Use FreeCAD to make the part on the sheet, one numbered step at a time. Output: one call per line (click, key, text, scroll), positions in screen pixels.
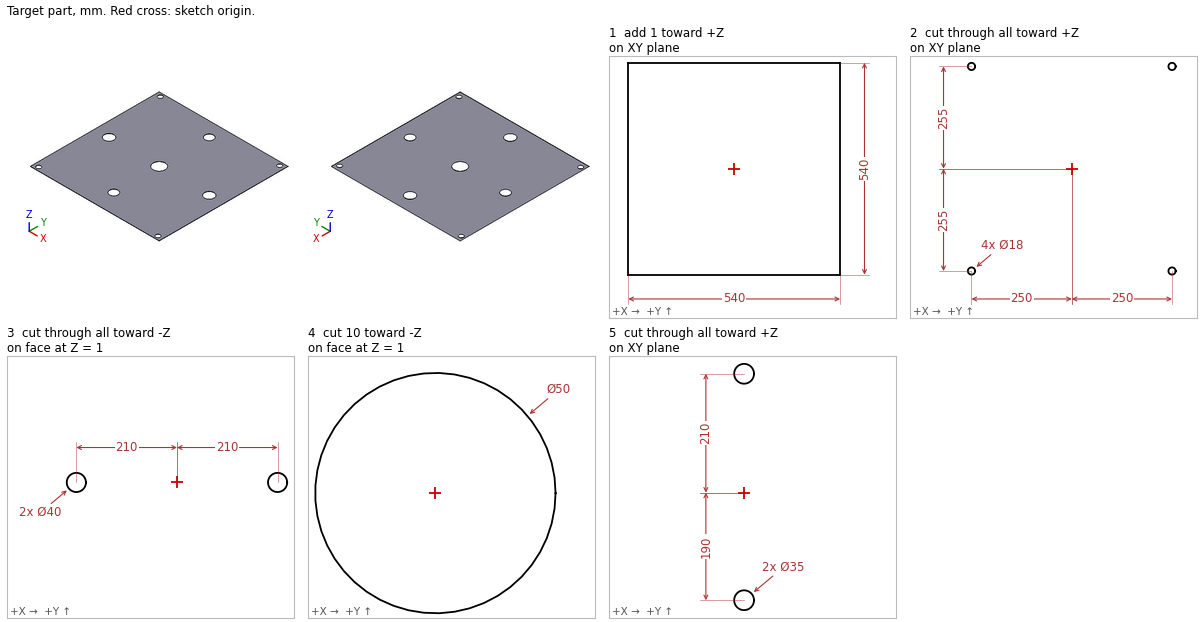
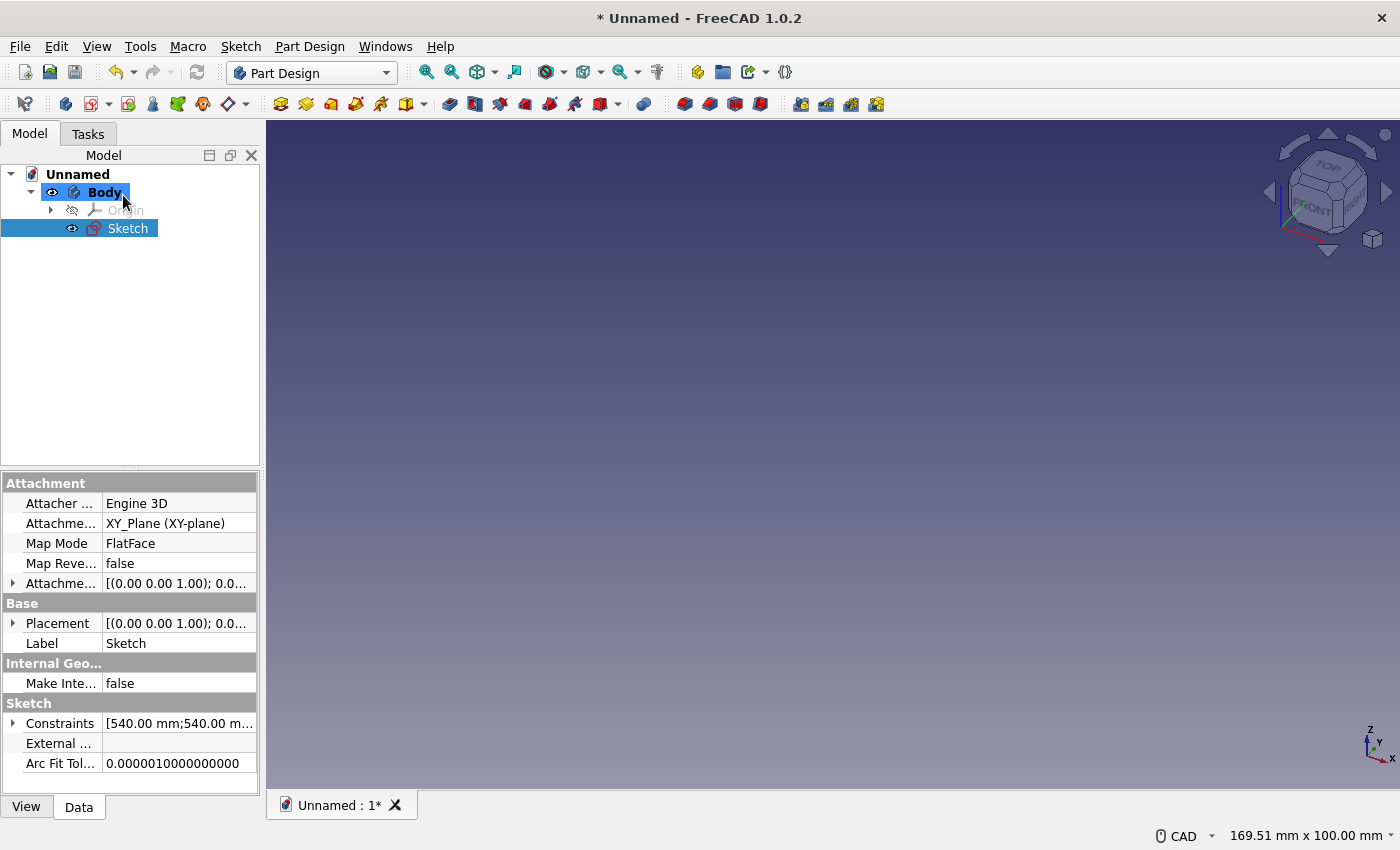
click(281, 104)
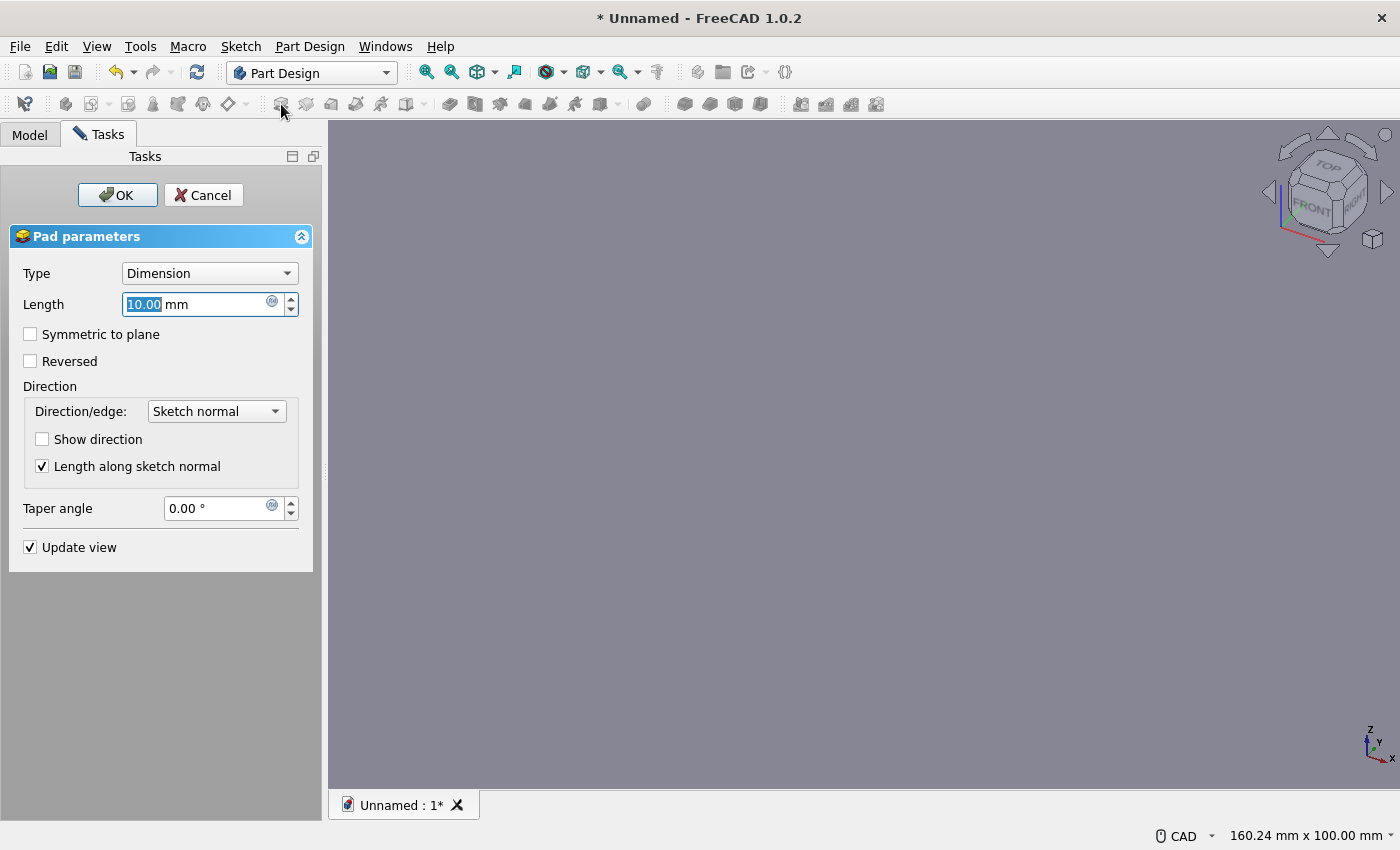
text(1)
key(Tab)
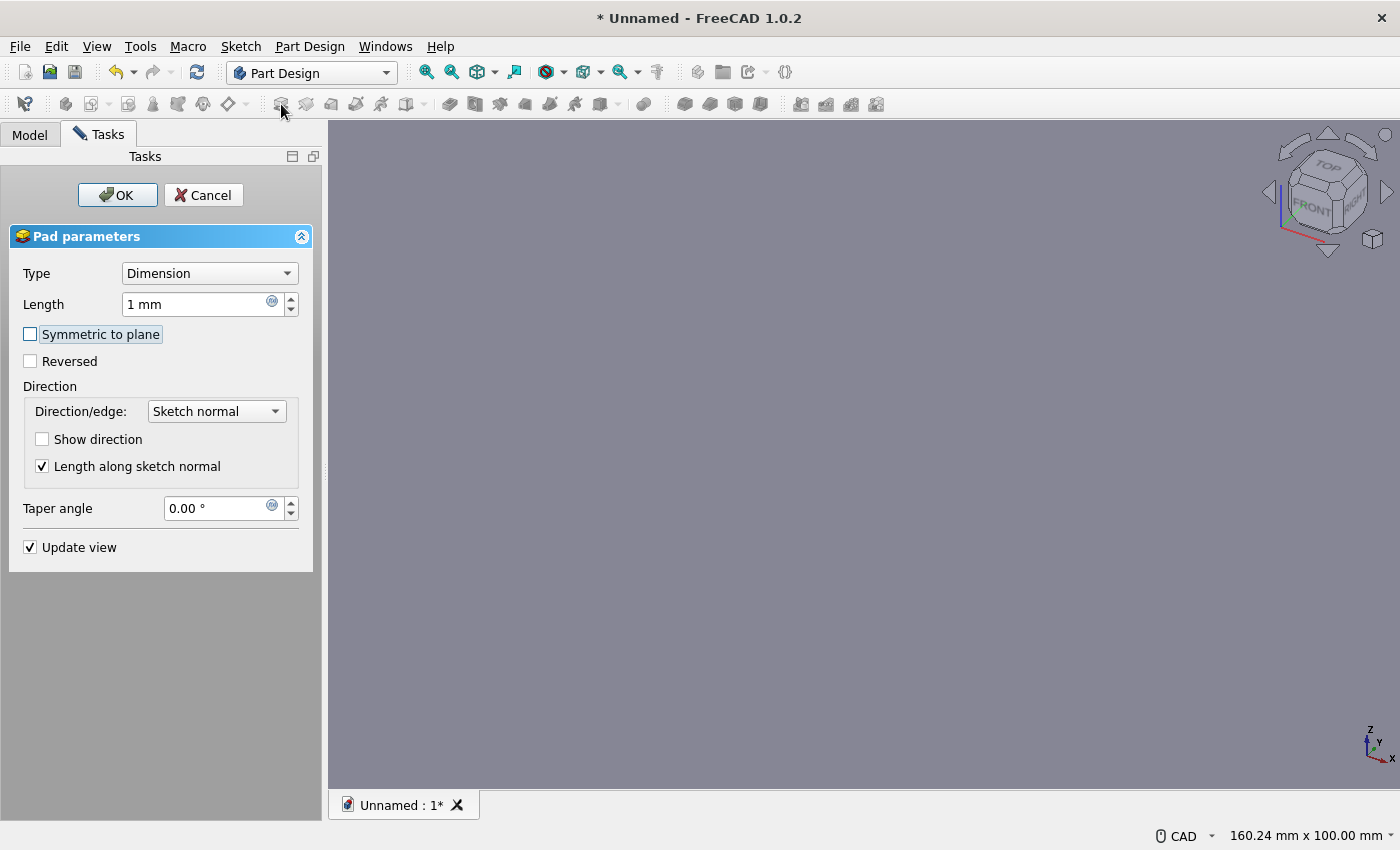
click(118, 195)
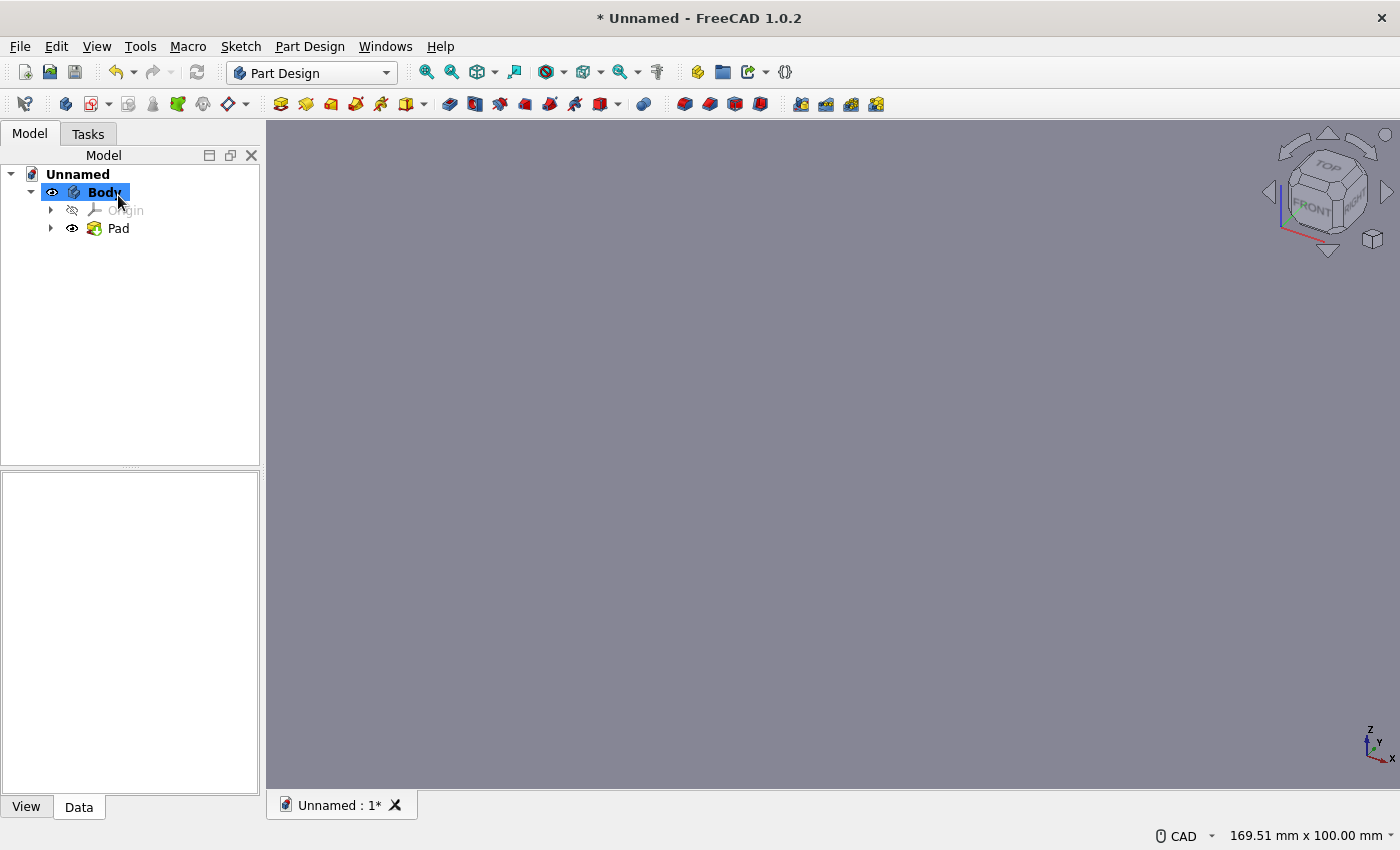
click(427, 72)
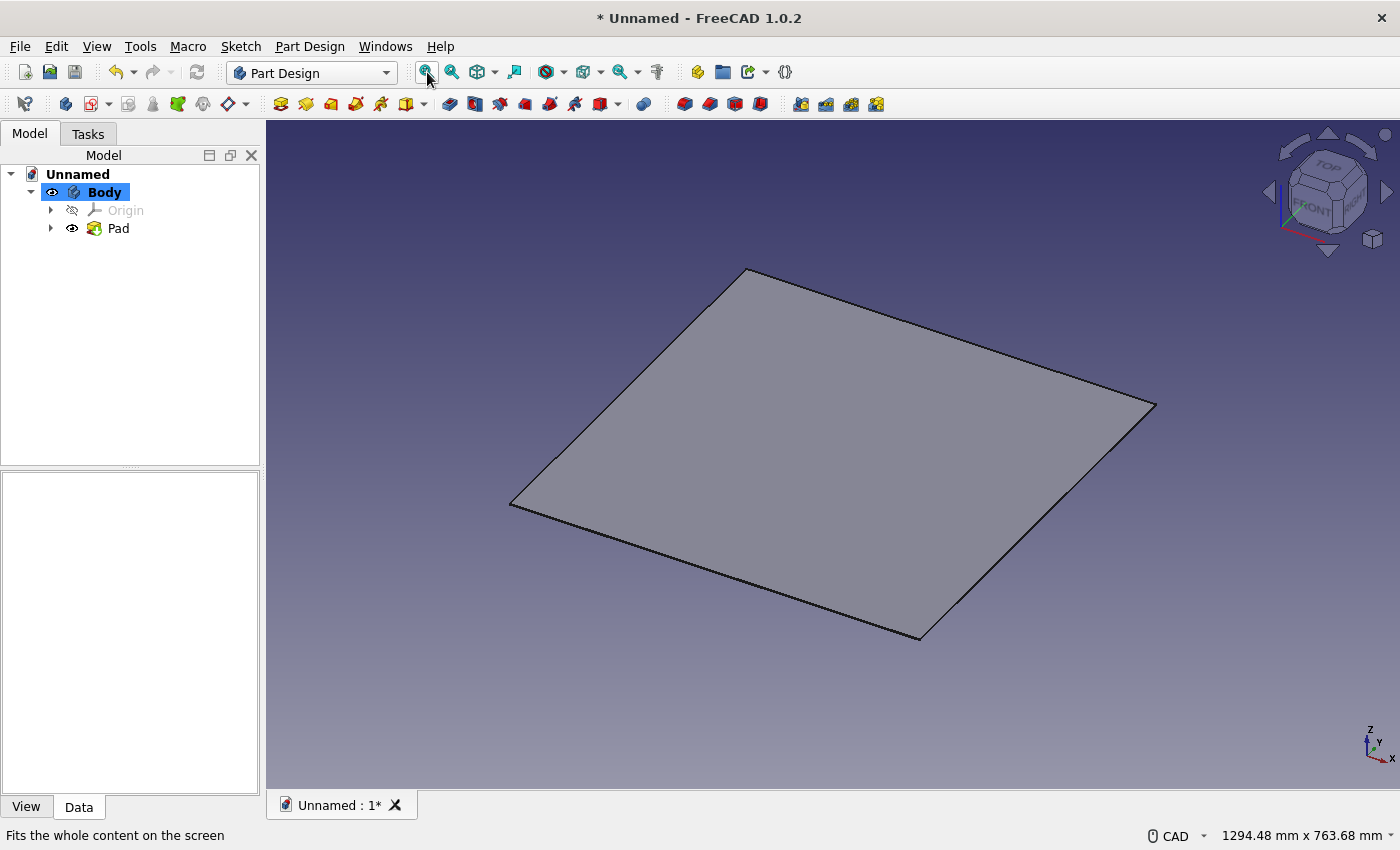
click(90, 104)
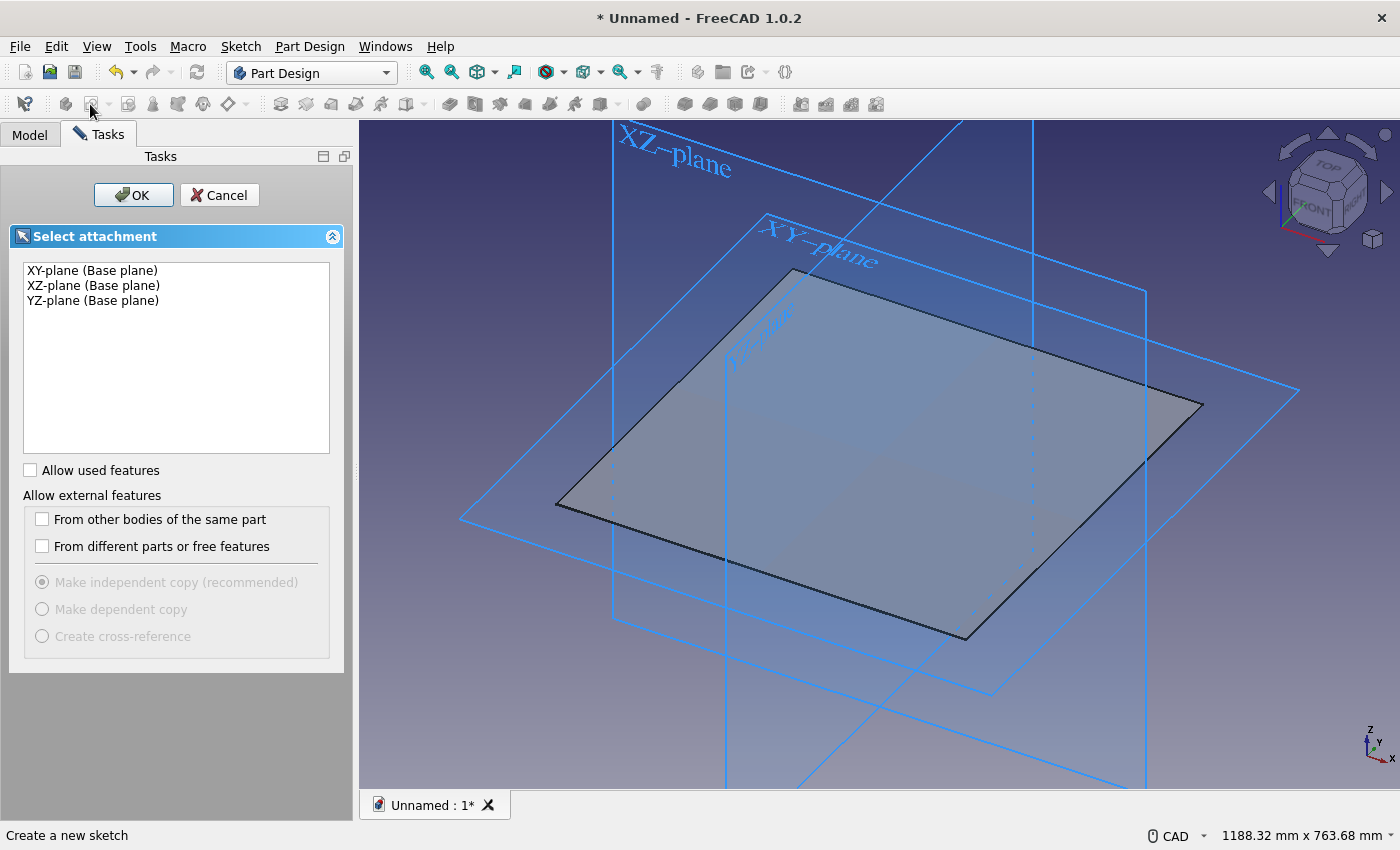
click(84, 270)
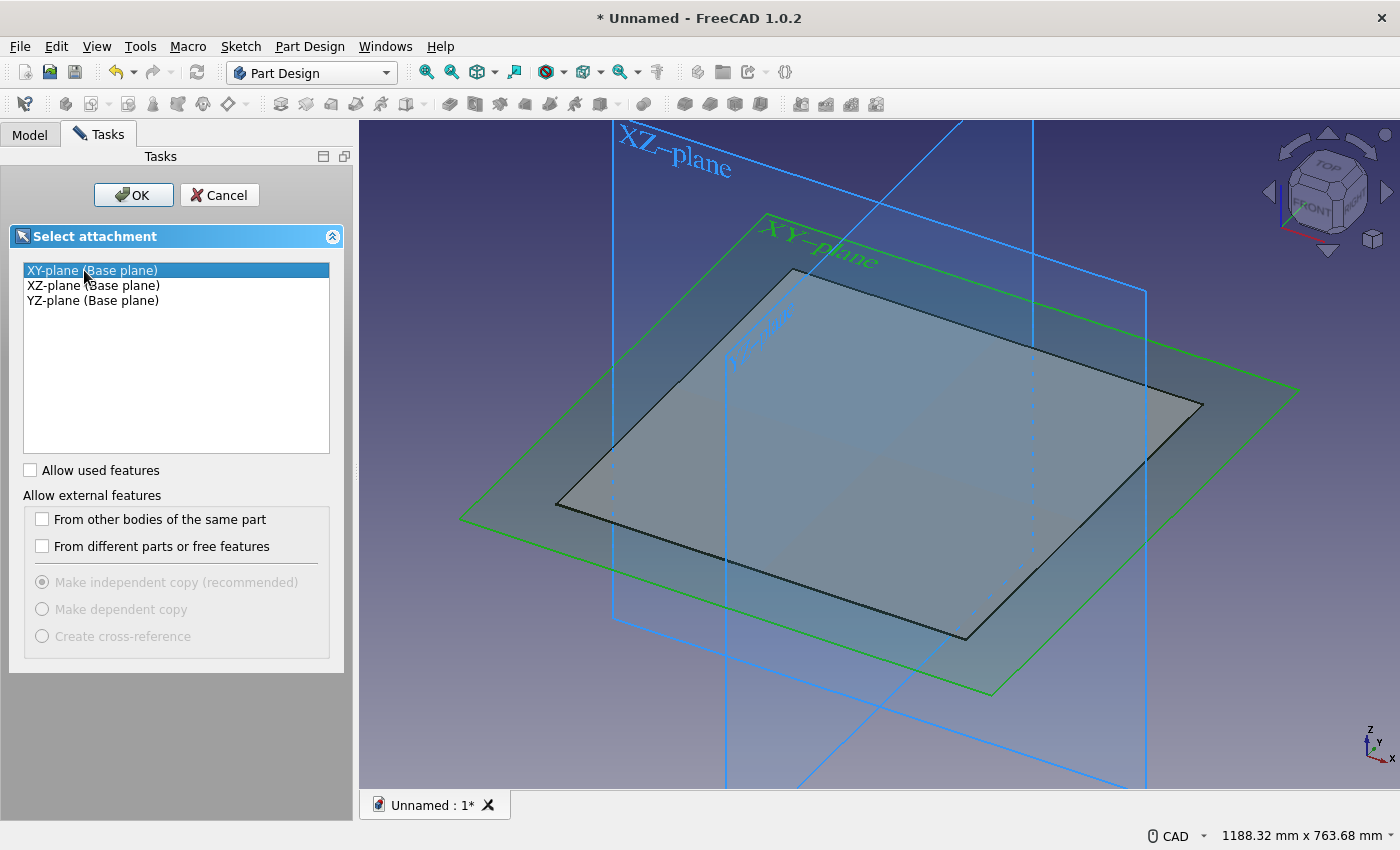
click(134, 195)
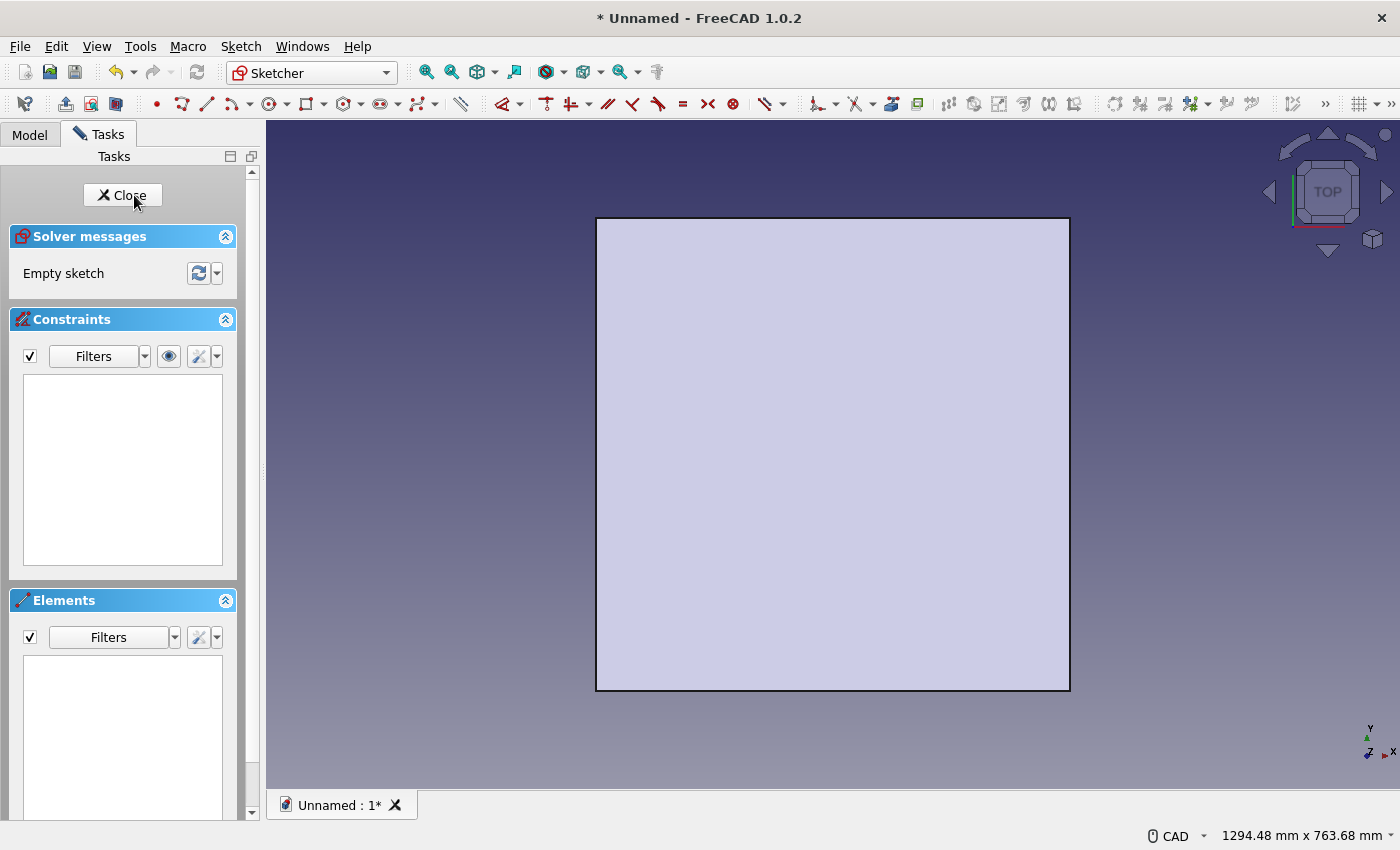
key(q)
key(s)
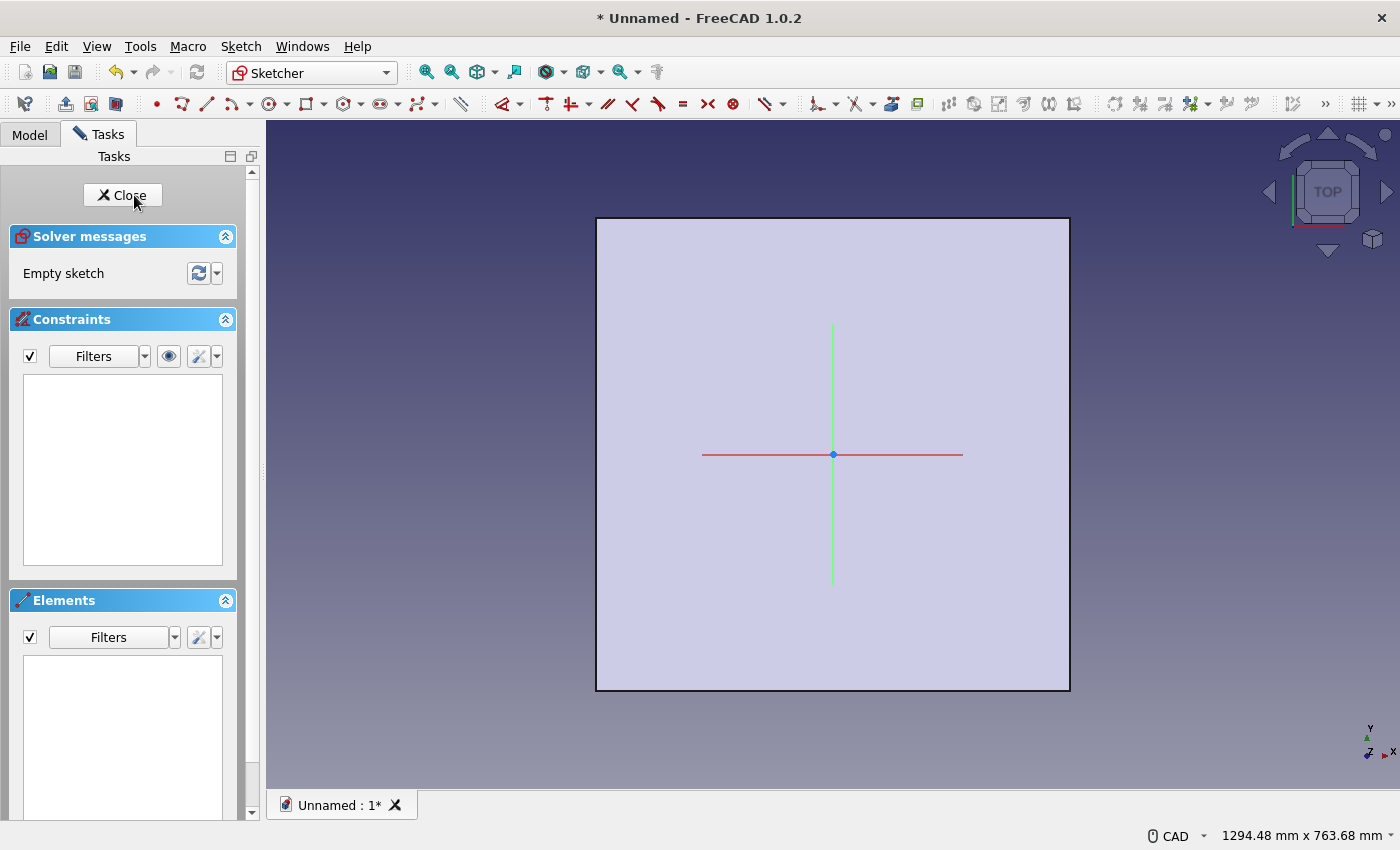
key(g)
key(c)